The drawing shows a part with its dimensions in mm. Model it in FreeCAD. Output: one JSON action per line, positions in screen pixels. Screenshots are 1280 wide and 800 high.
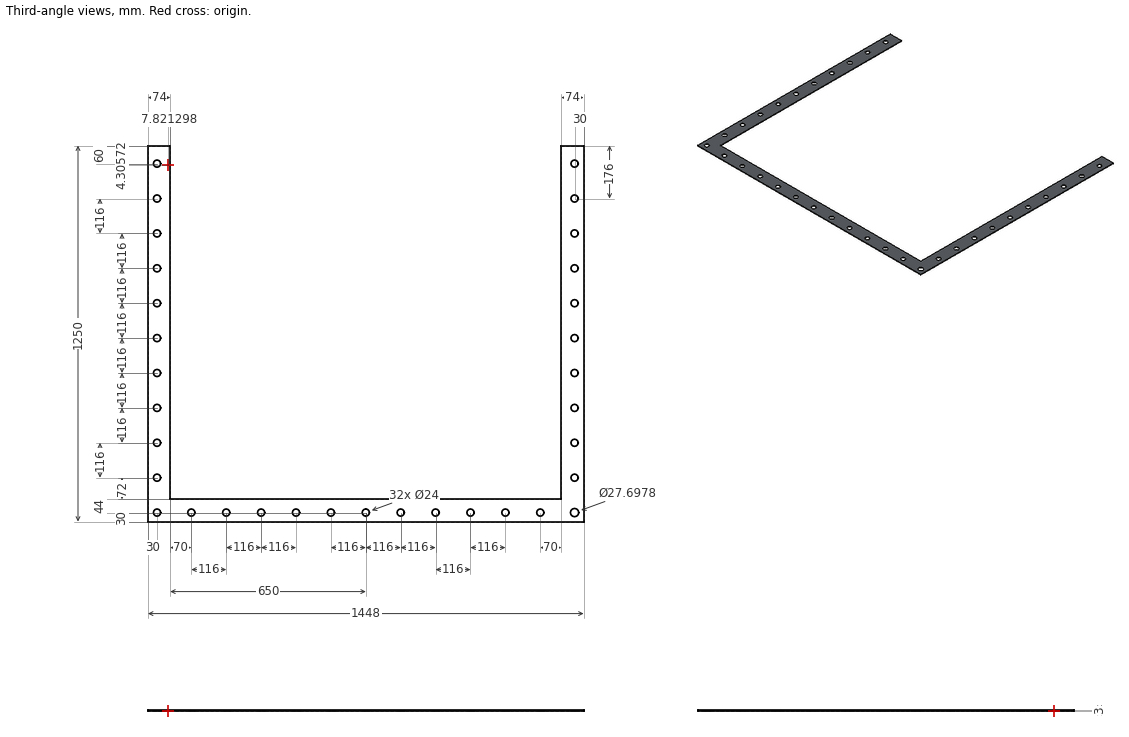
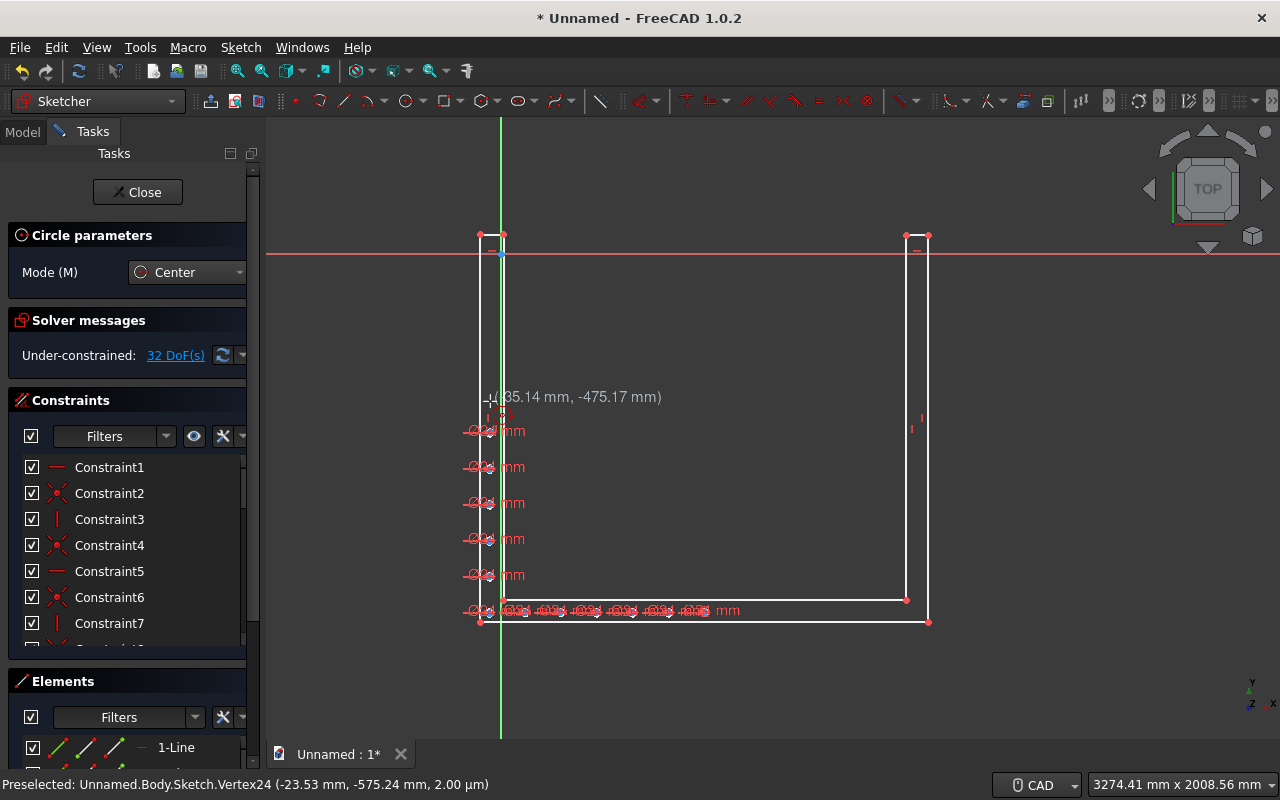
{"action": "scroll", "coordinate": [490, 397], "scroll_direction": "up", "scroll_amount": 3}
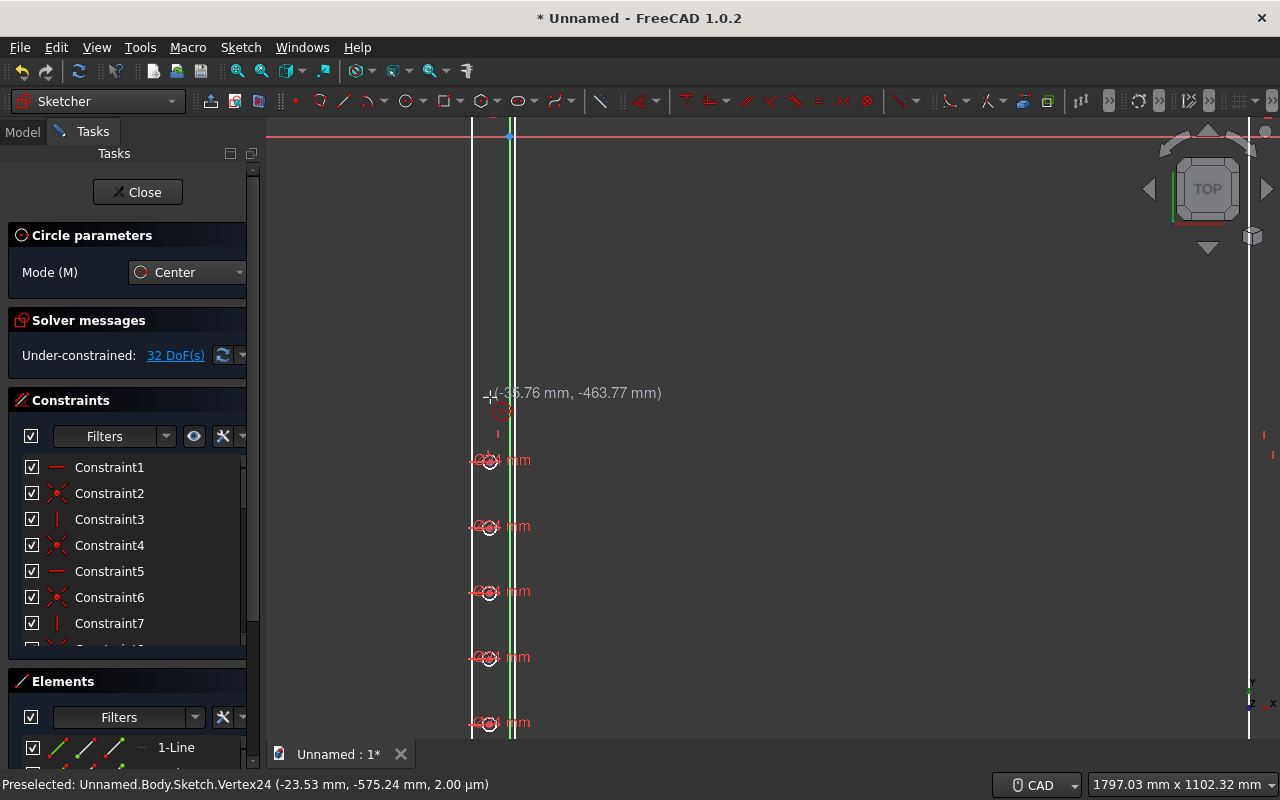
{"action": "left_click", "coordinate": [490, 396]}
{"action": "mouse_move", "coordinate": [494, 391]}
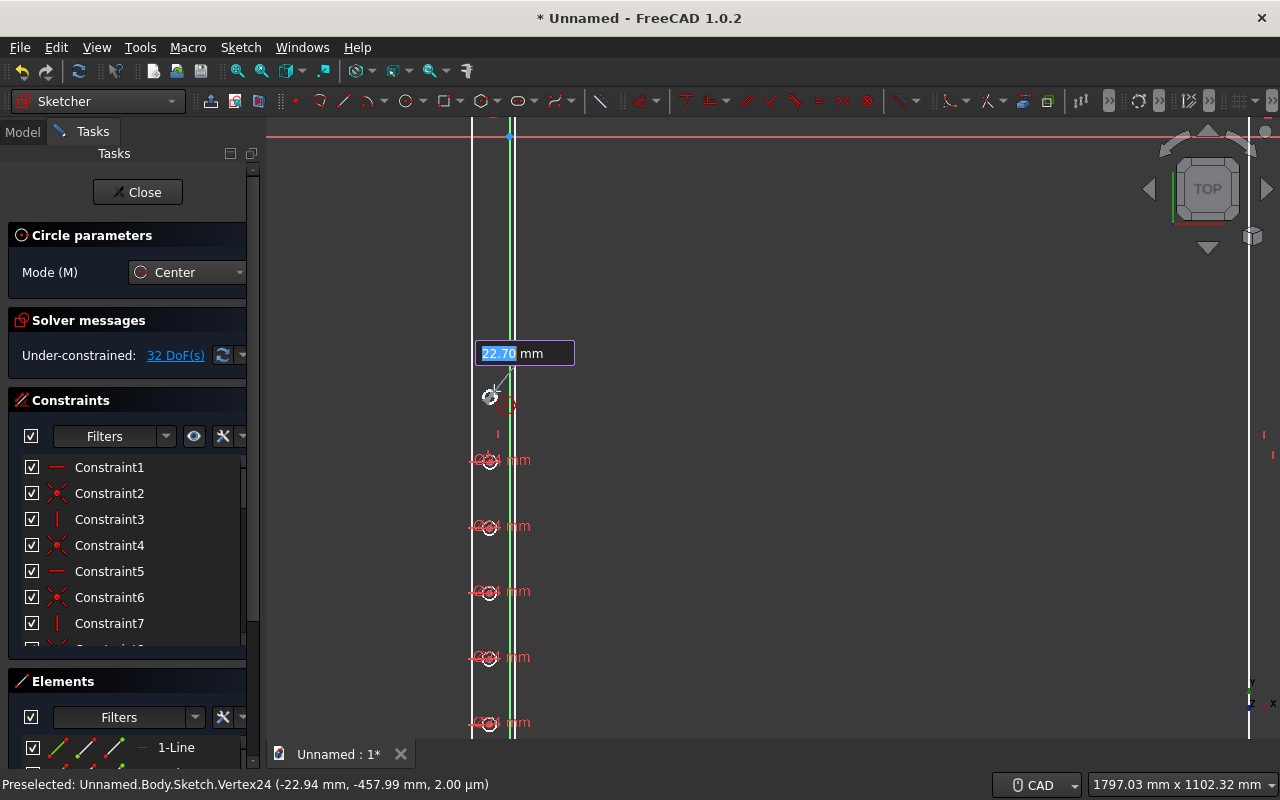
{"action": "type", "text": "24"}
{"action": "key", "text": "Return"}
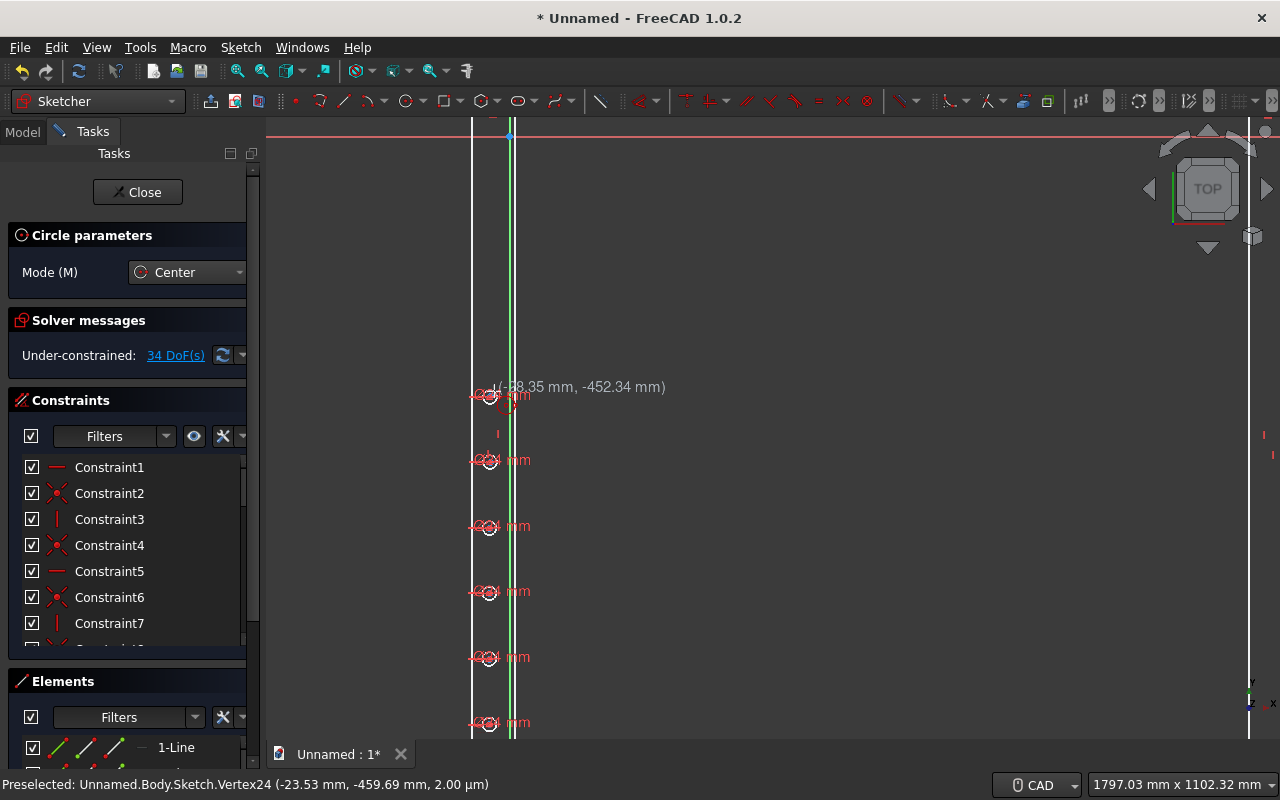
{"action": "scroll", "coordinate": [490, 331], "scroll_direction": "up", "scroll_amount": 7}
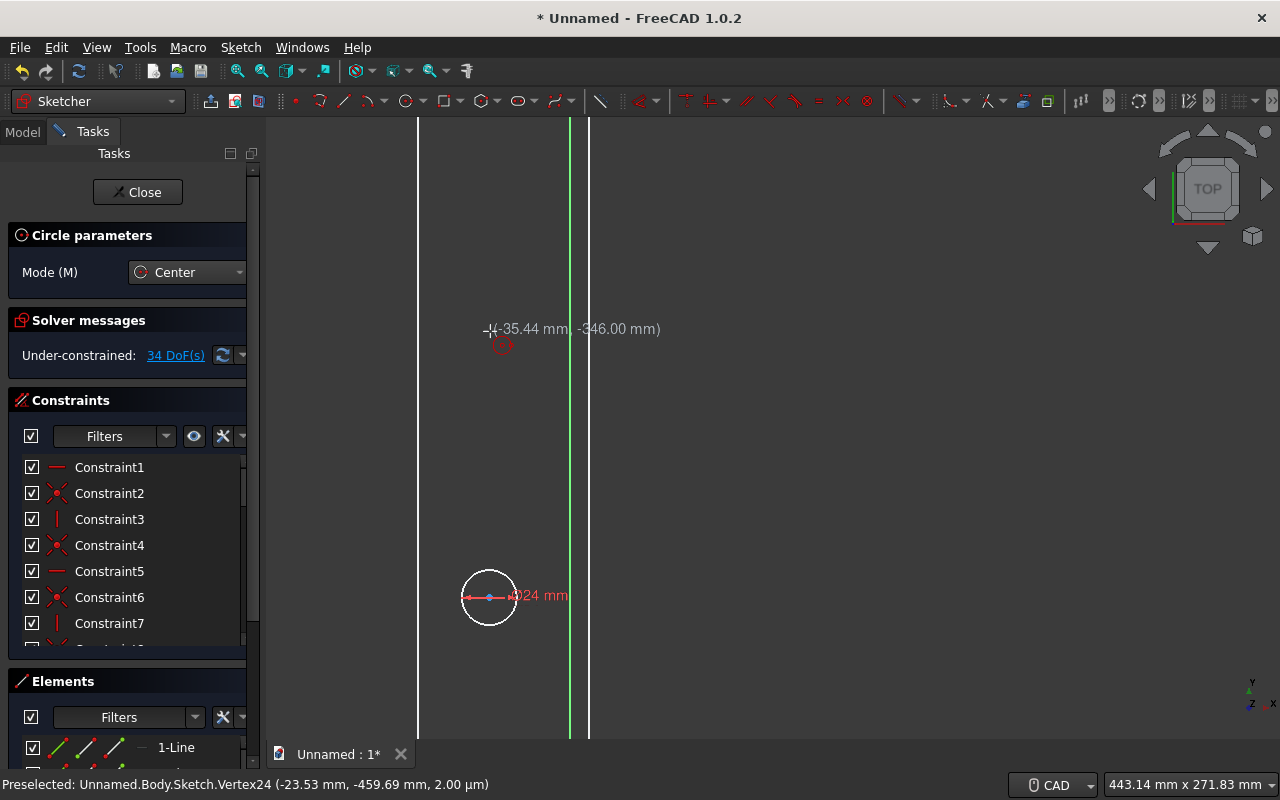
{"action": "scroll", "coordinate": [490, 366], "scroll_direction": "down", "scroll_amount": 10}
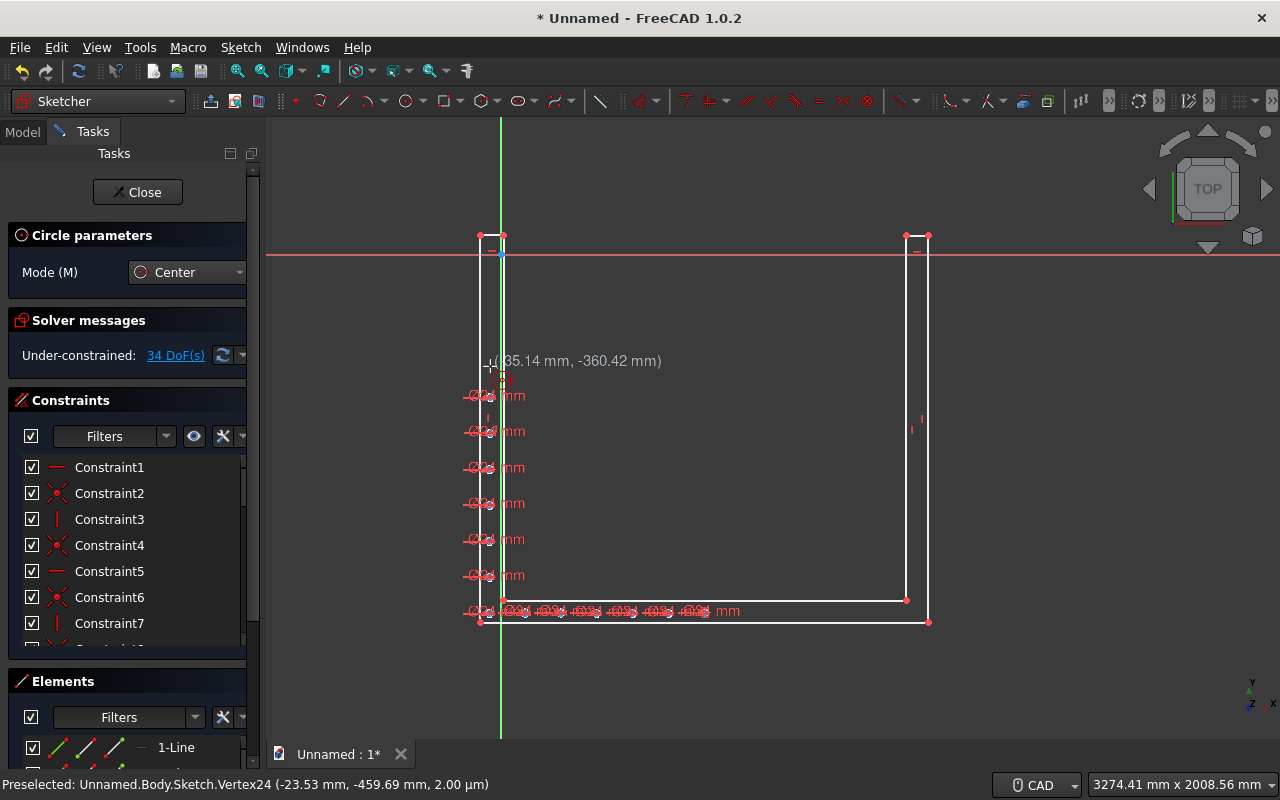
{"action": "scroll", "coordinate": [490, 361], "scroll_direction": "up", "scroll_amount": 3}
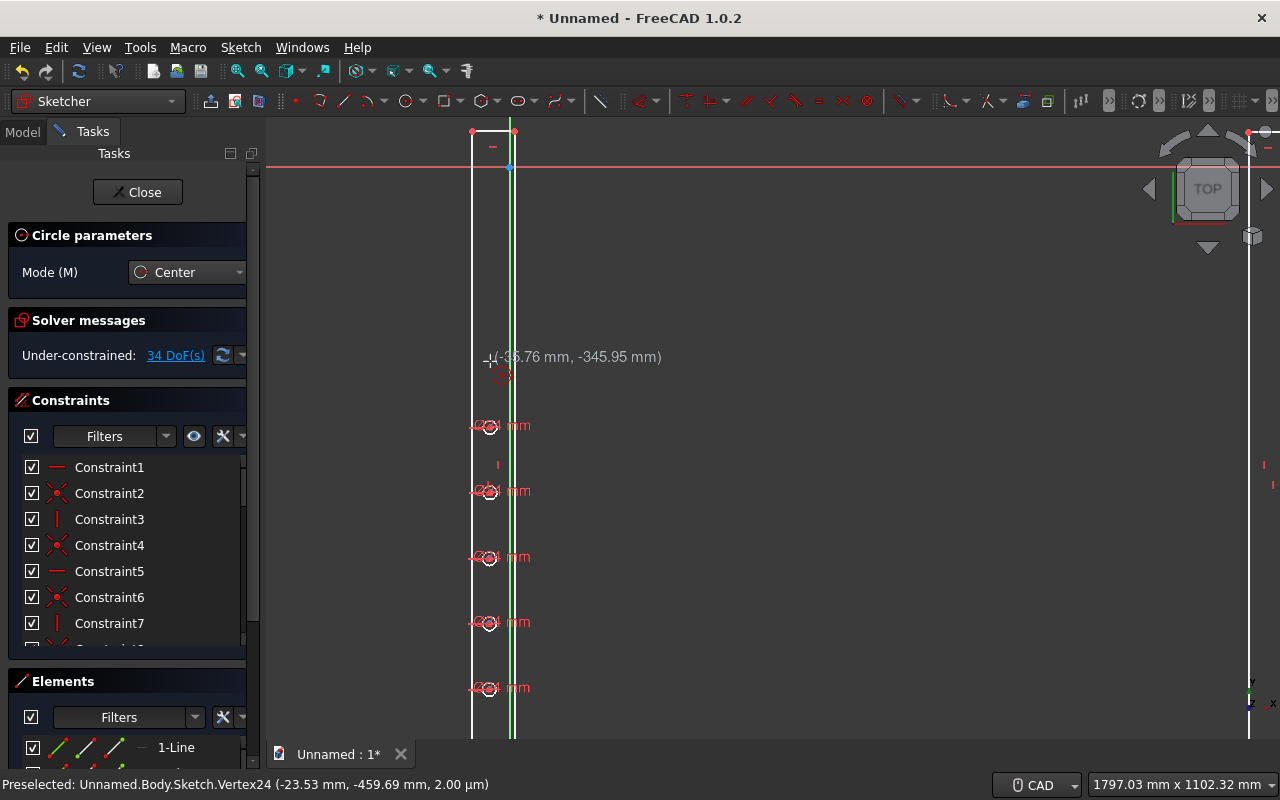
{"action": "left_click", "coordinate": [490, 361]}
{"action": "mouse_move", "coordinate": [494, 356]}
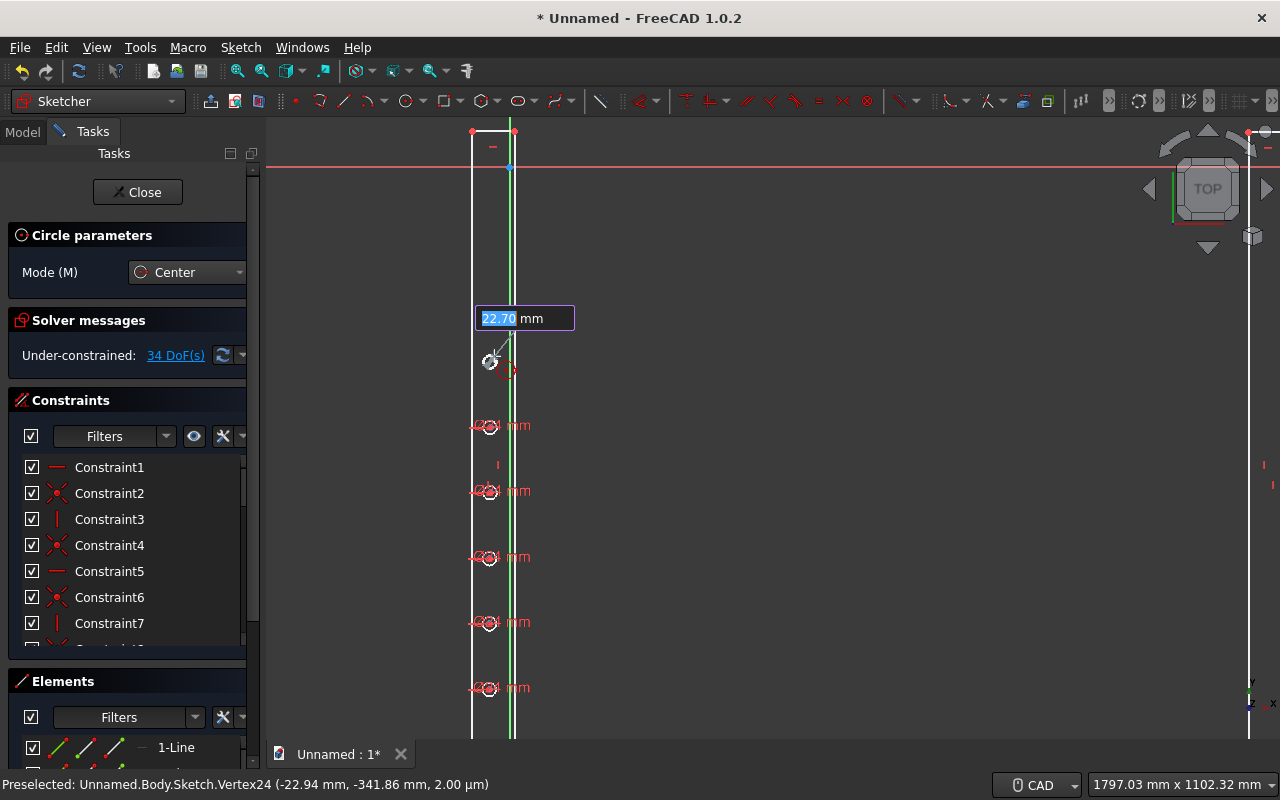
{"action": "type", "text": "24"}
{"action": "key", "text": "Return"}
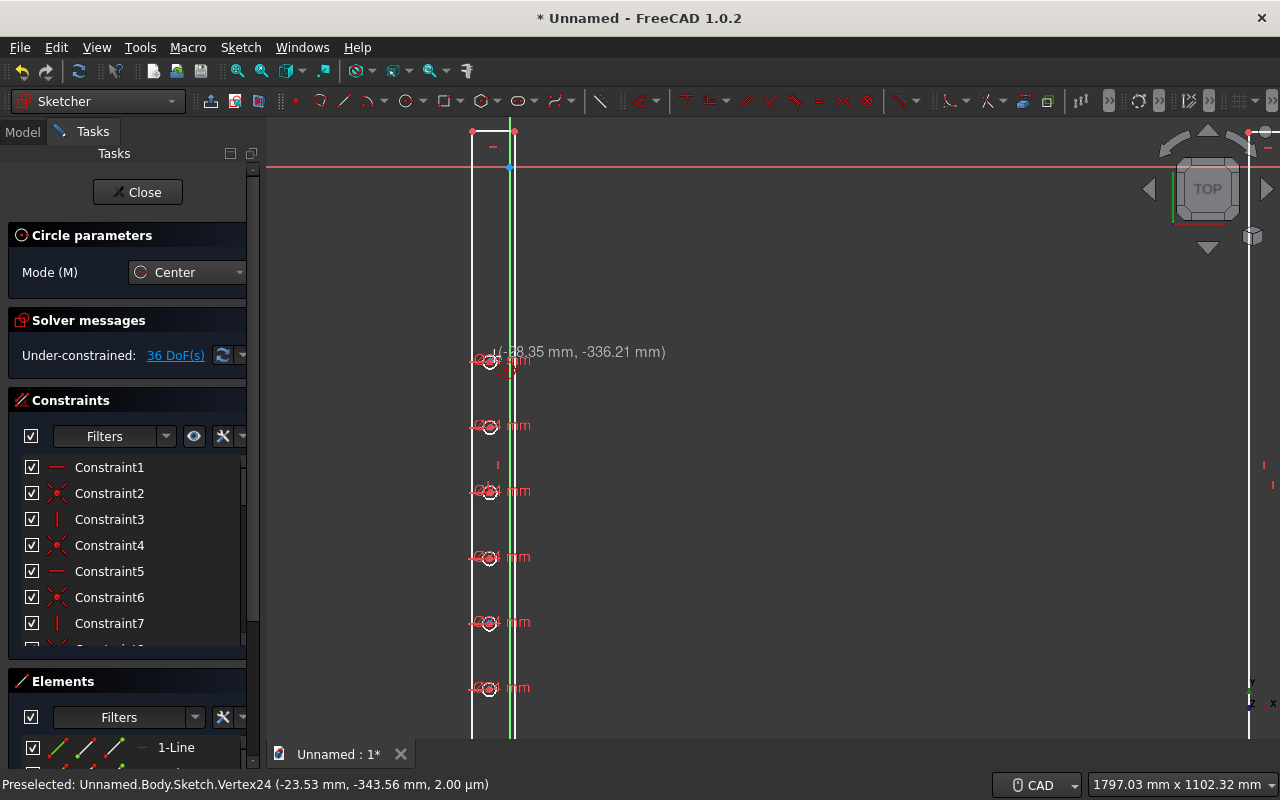
{"action": "scroll", "coordinate": [490, 296], "scroll_direction": "up", "scroll_amount": 7}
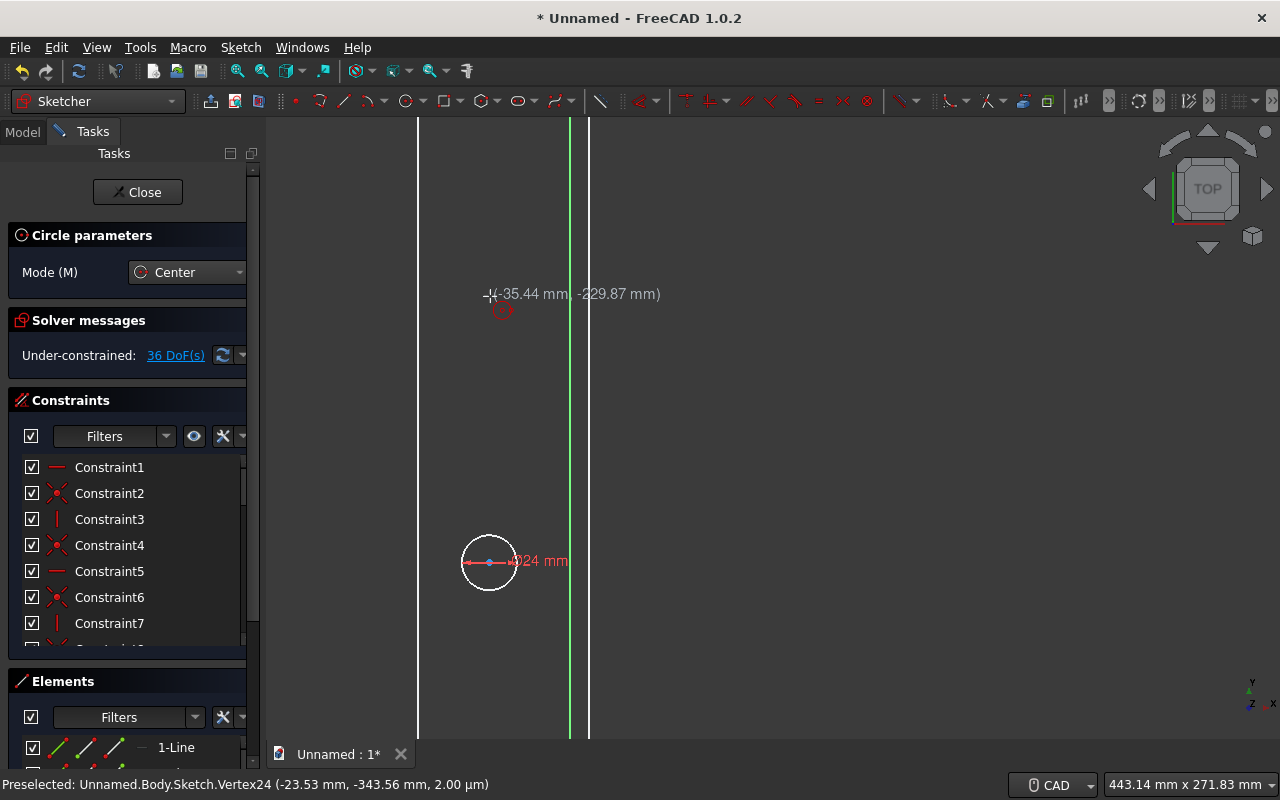
{"action": "scroll", "coordinate": [490, 330], "scroll_direction": "down", "scroll_amount": 10}